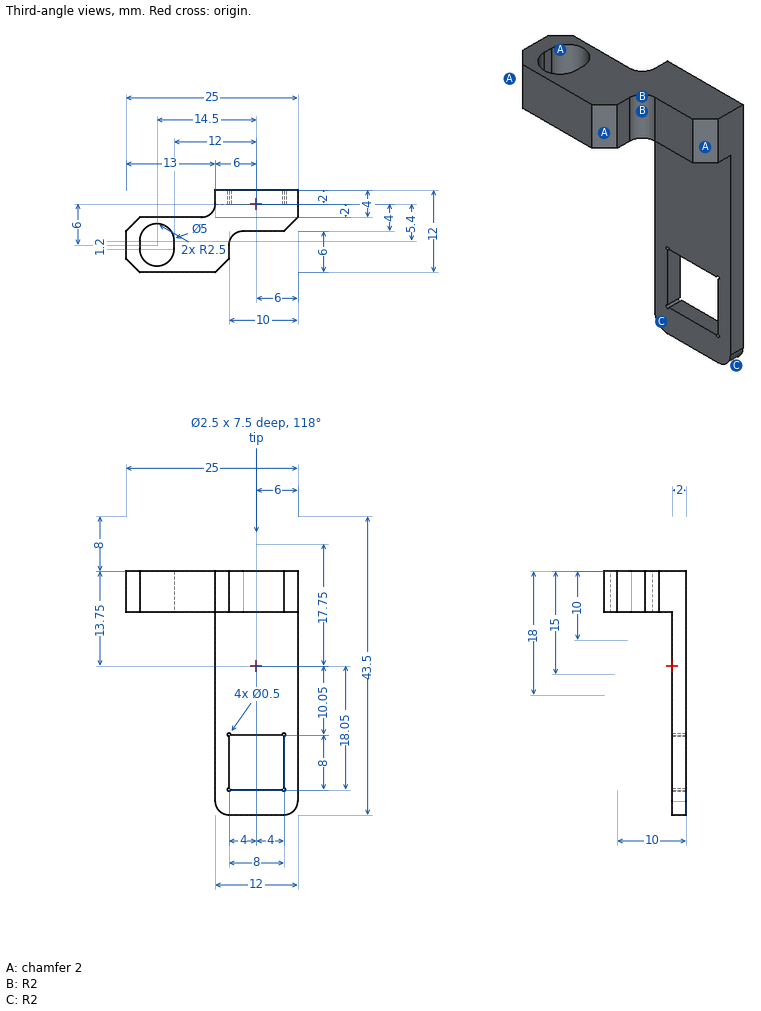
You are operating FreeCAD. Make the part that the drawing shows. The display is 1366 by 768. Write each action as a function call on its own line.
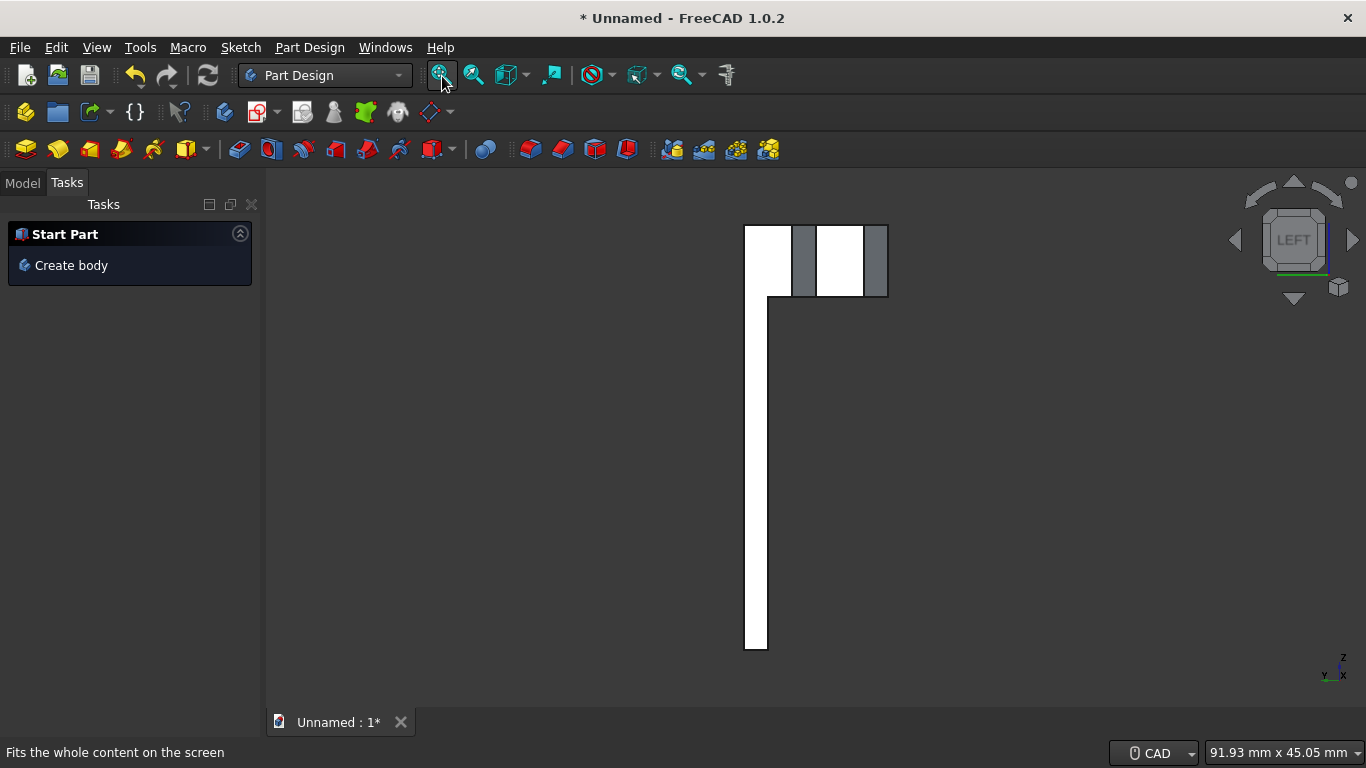
key(v)
key(3)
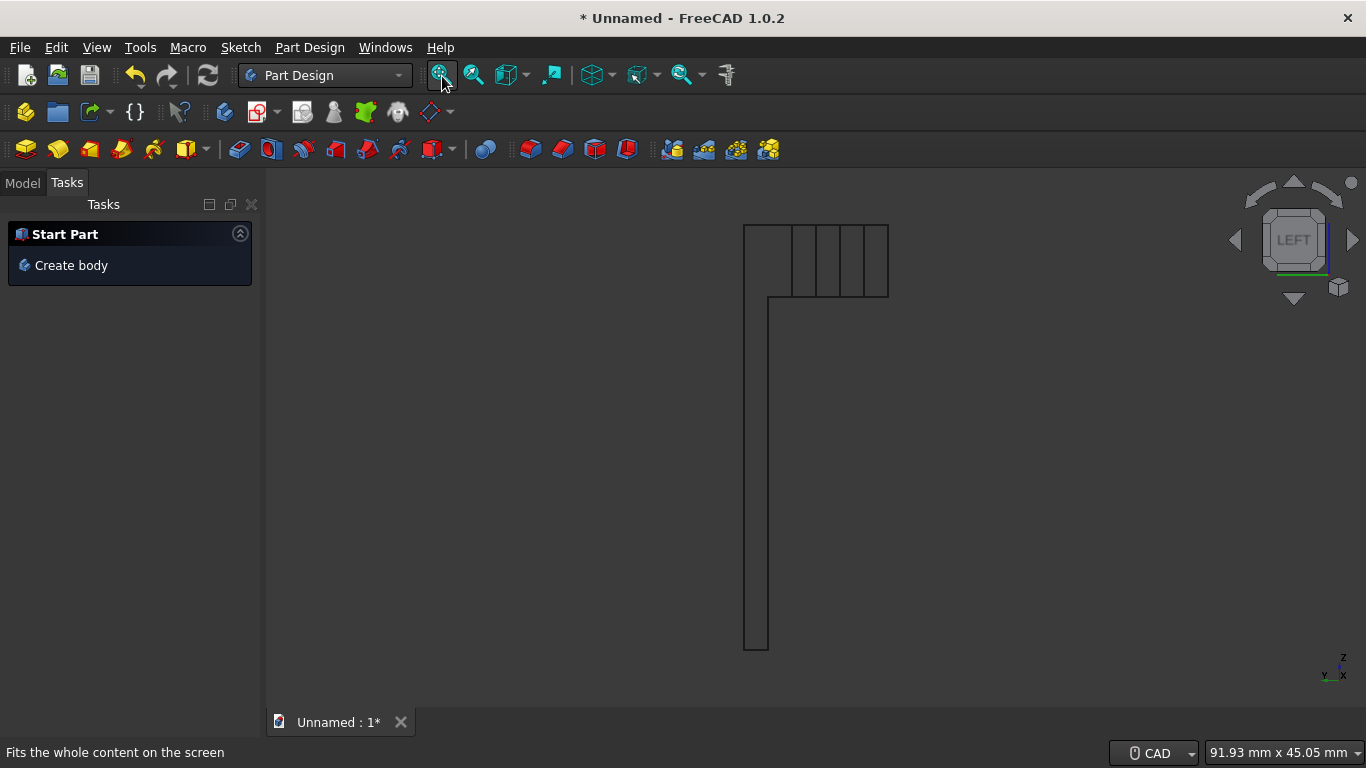
key(0)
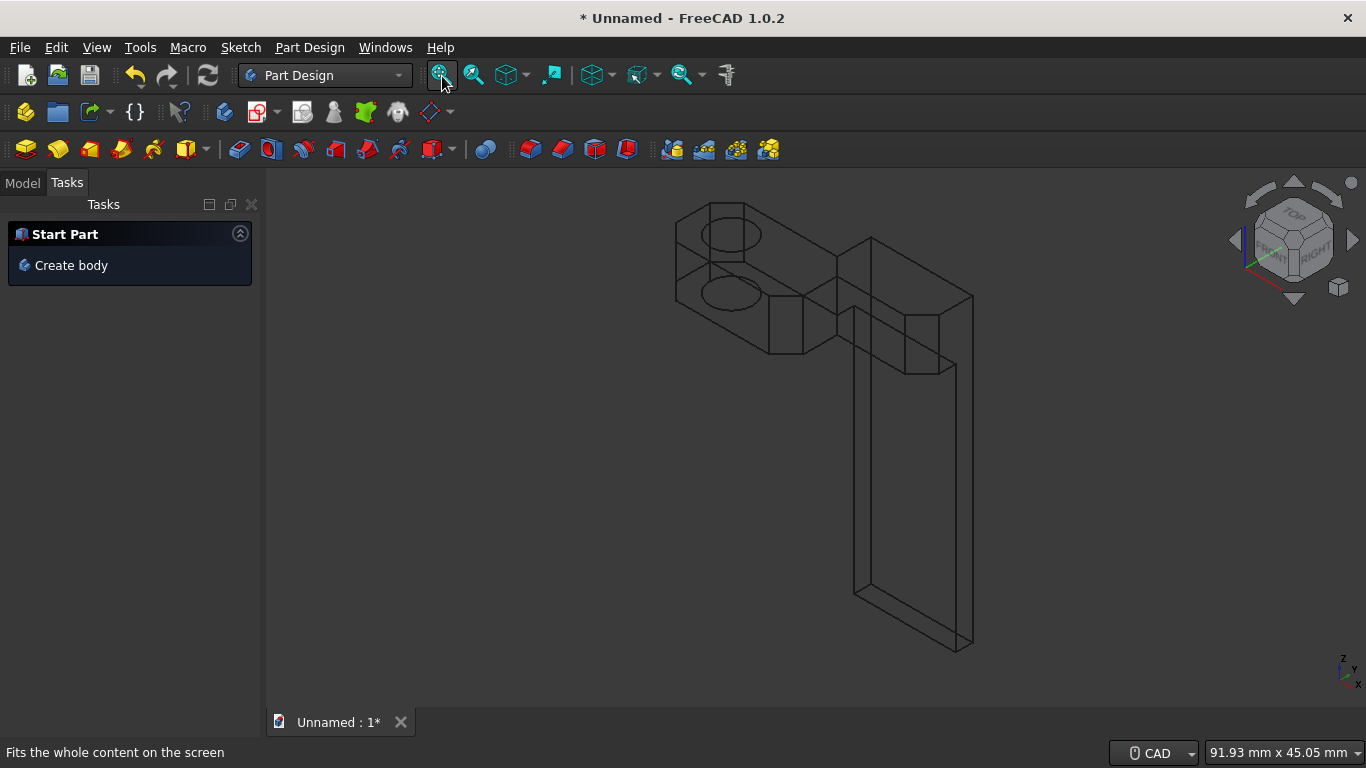
click(837, 305)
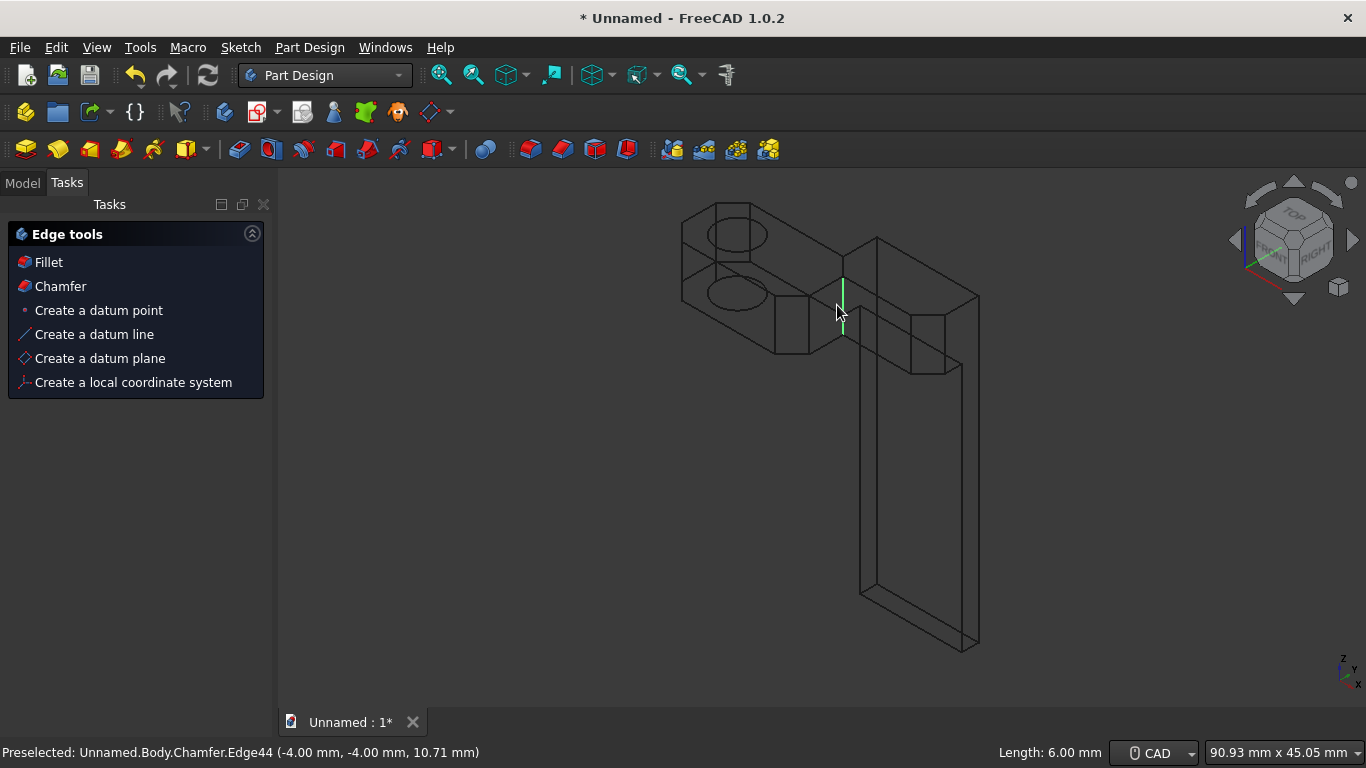
click(843, 267, ctrl)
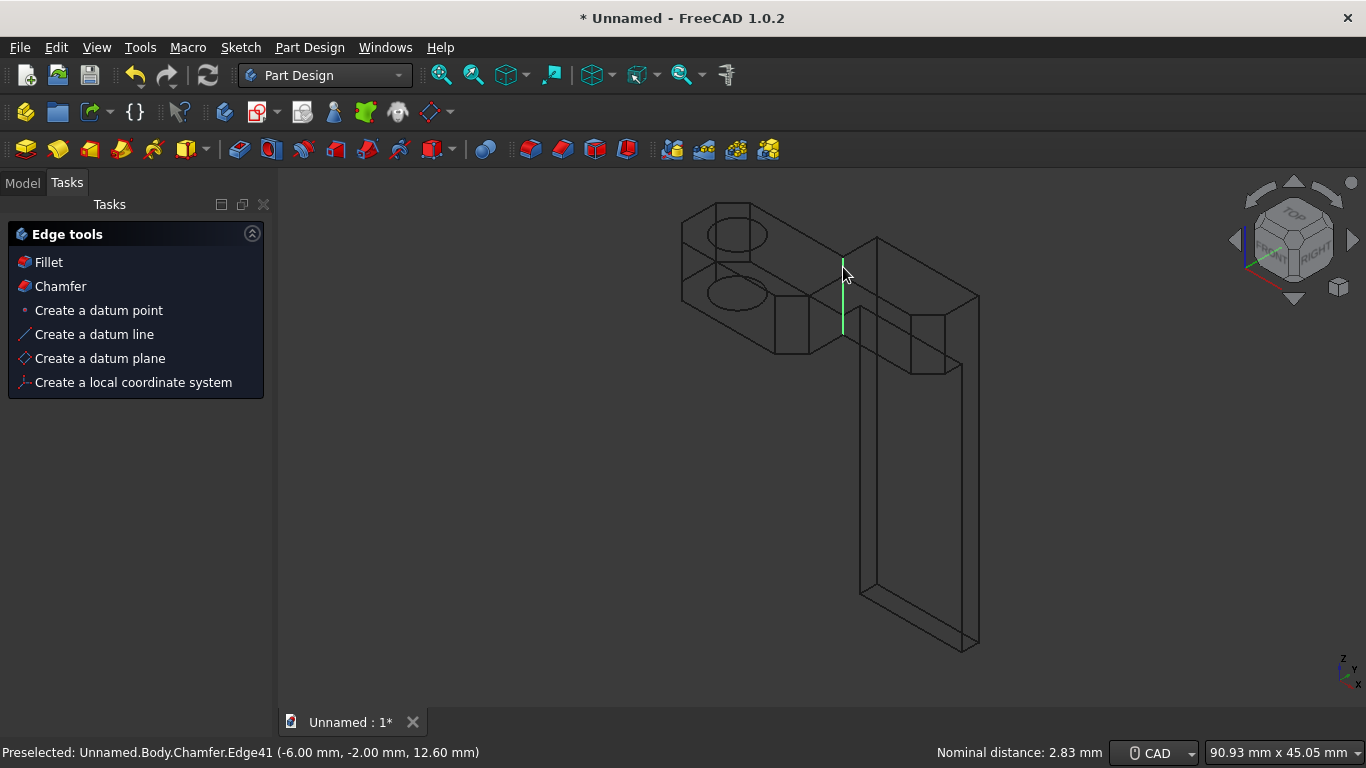
key(v)
key(1)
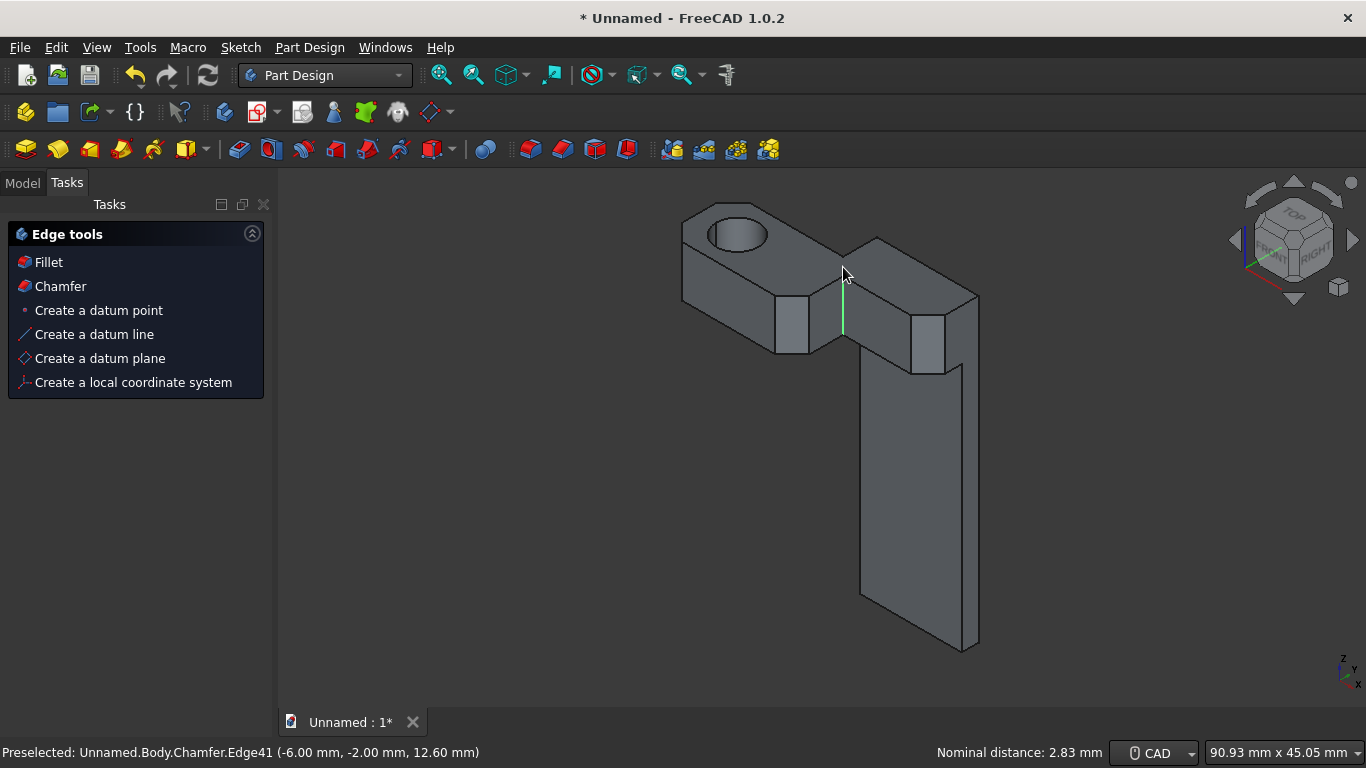
click(532, 150)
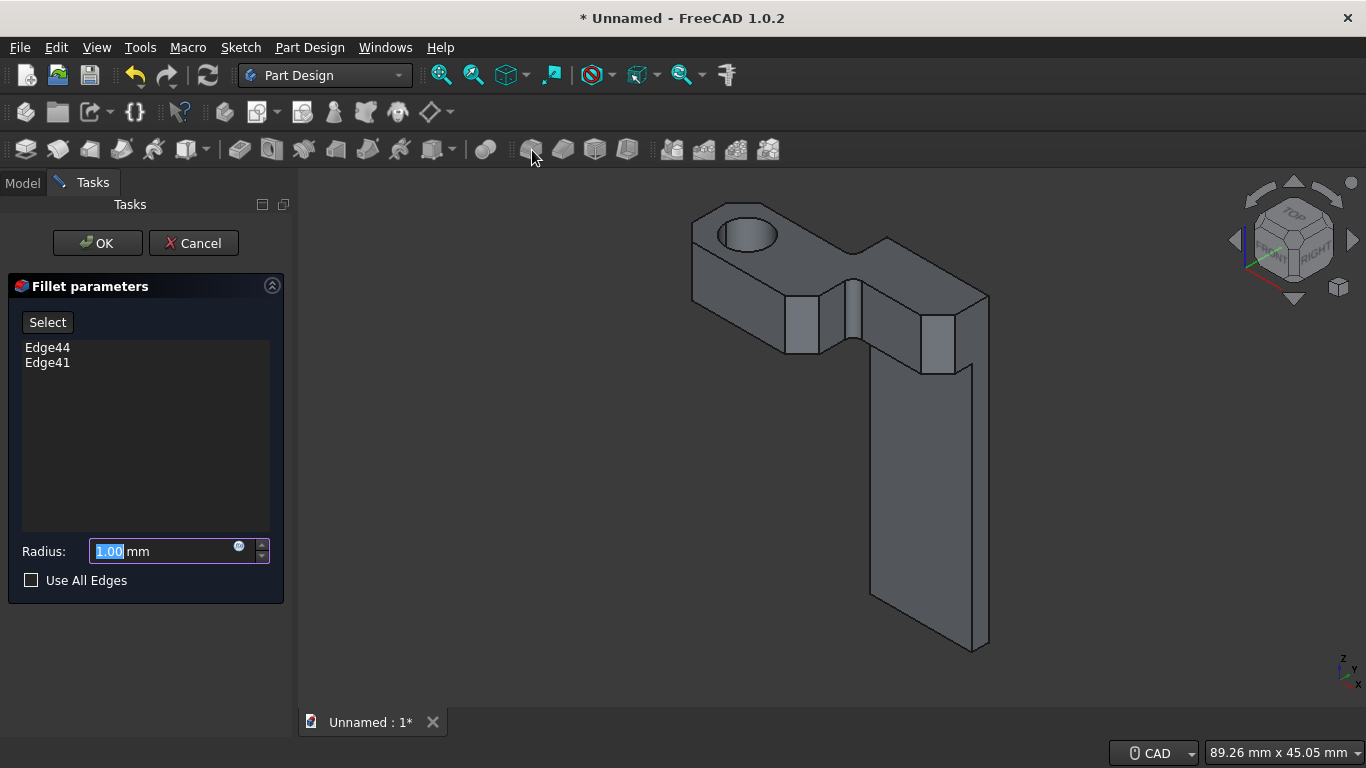
text(2)
key(Tab)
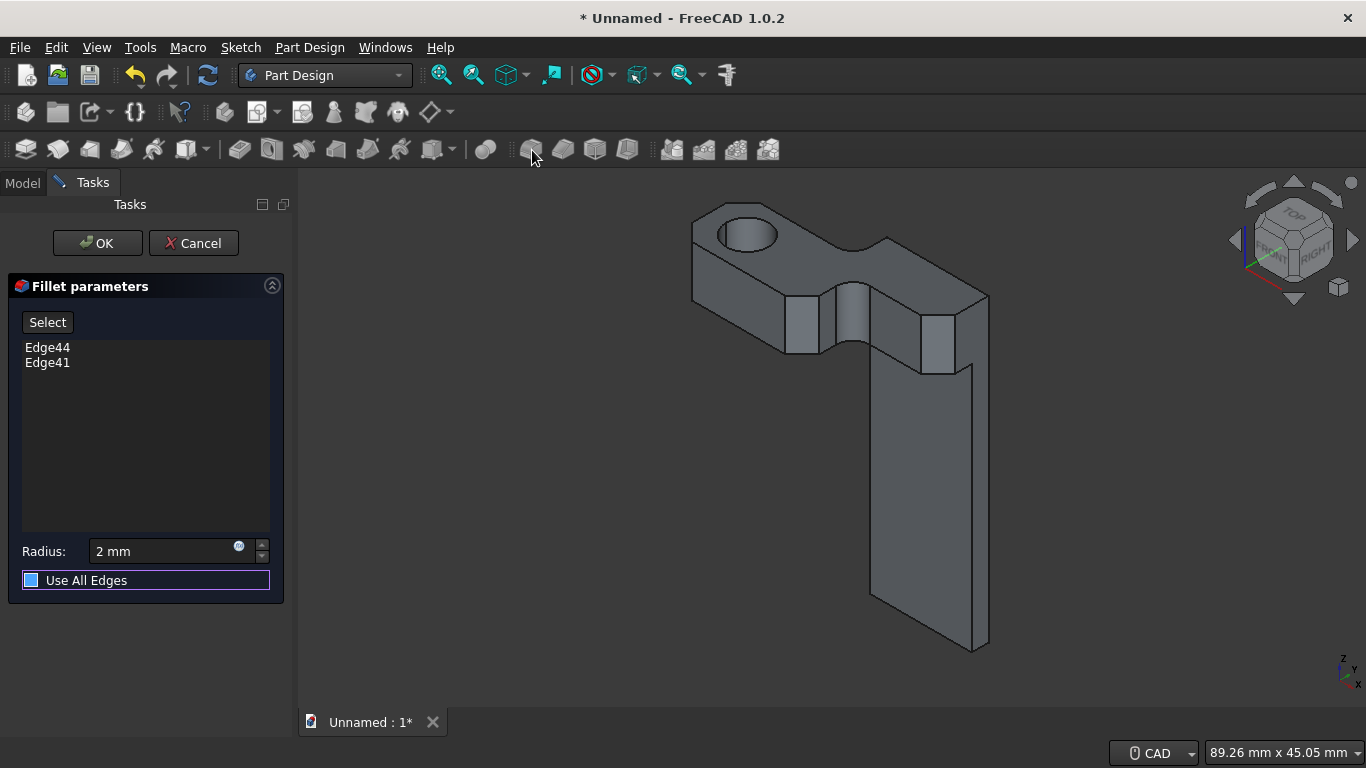
click(98, 243)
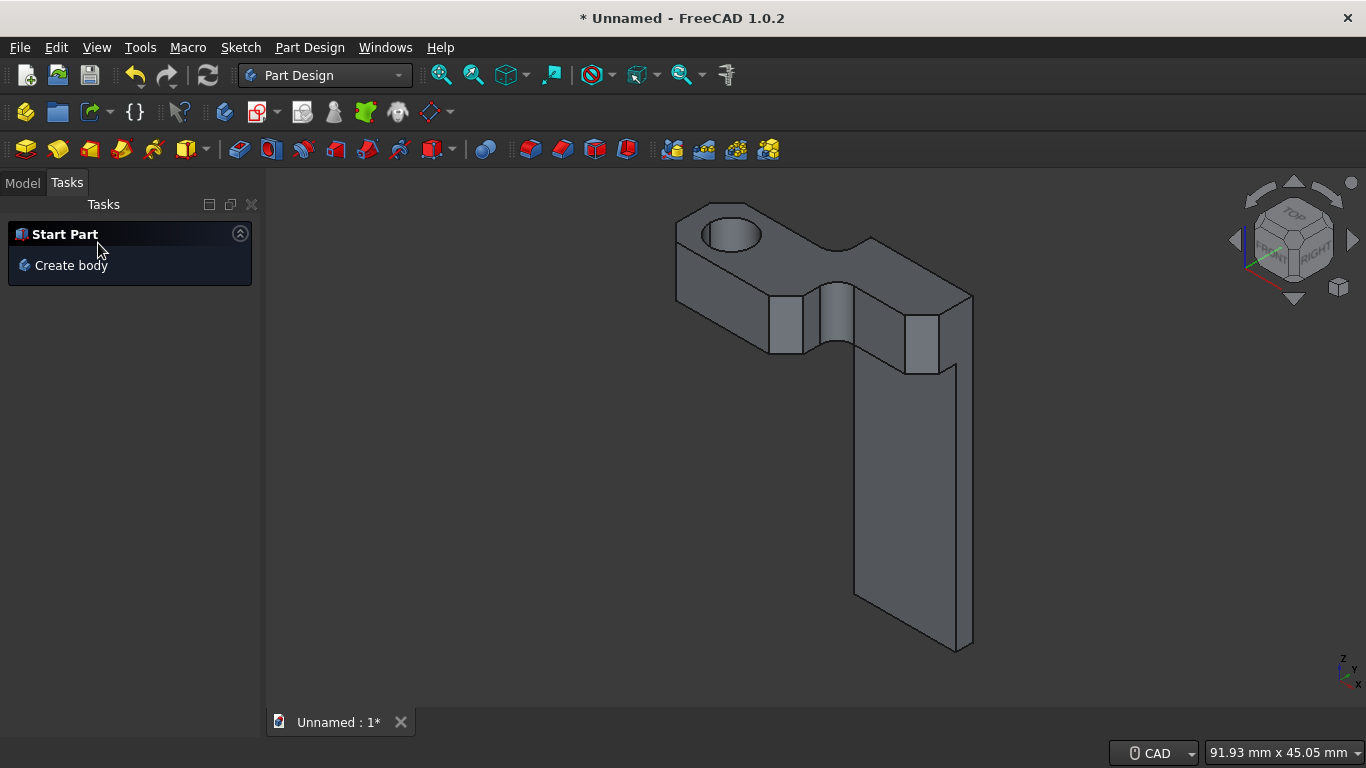
key(2)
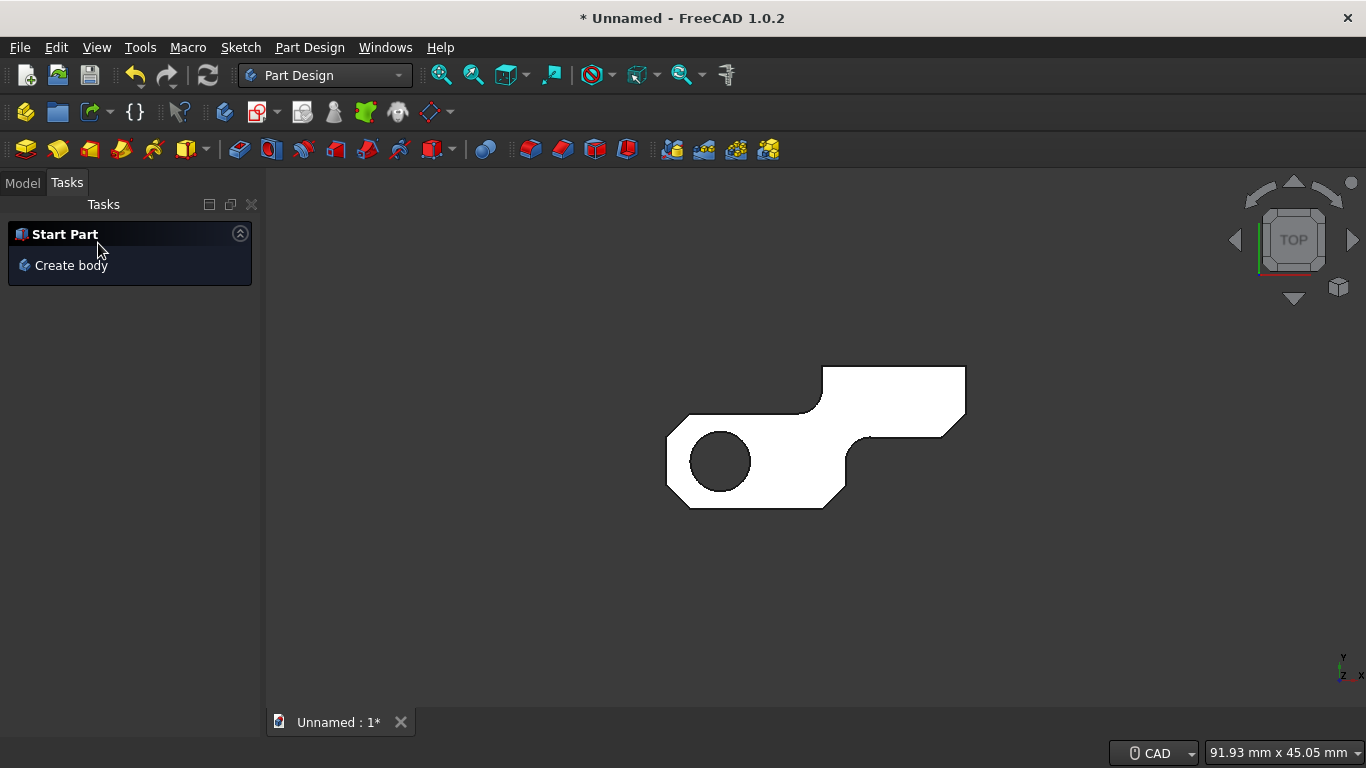
click(442, 76)